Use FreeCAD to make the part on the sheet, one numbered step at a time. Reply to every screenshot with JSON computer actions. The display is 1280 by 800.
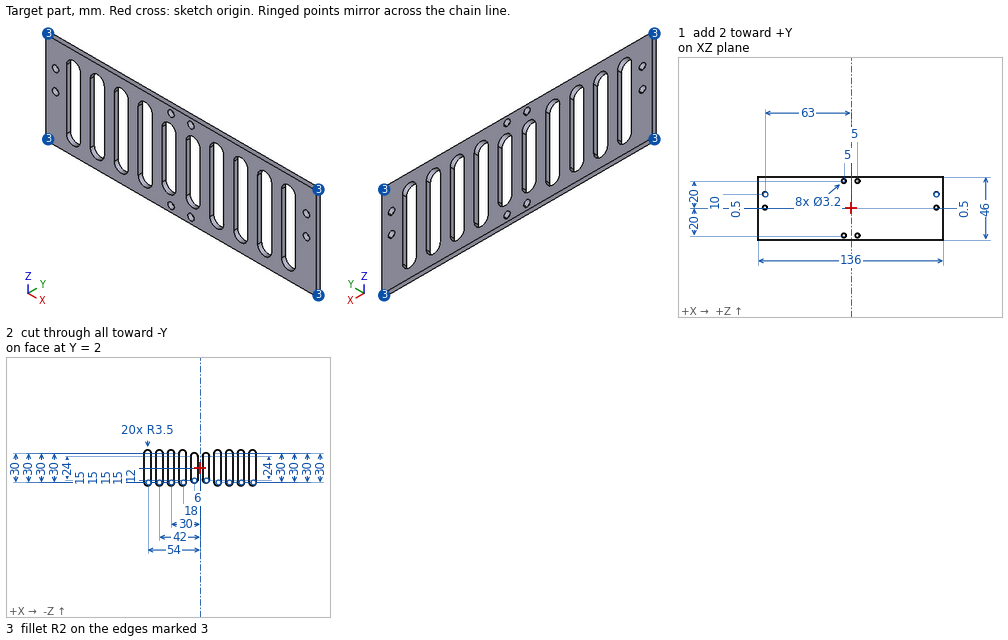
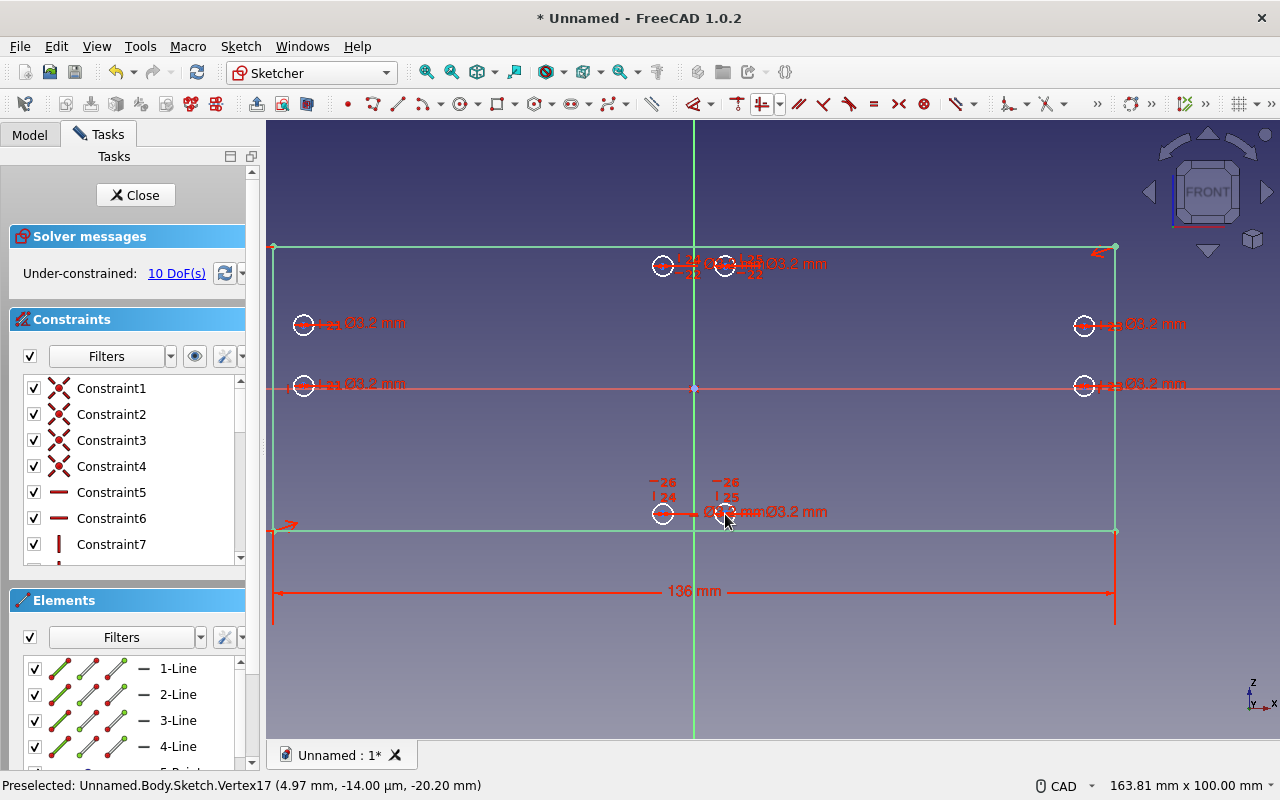
{"action": "left_click", "coordinate": [304, 325]}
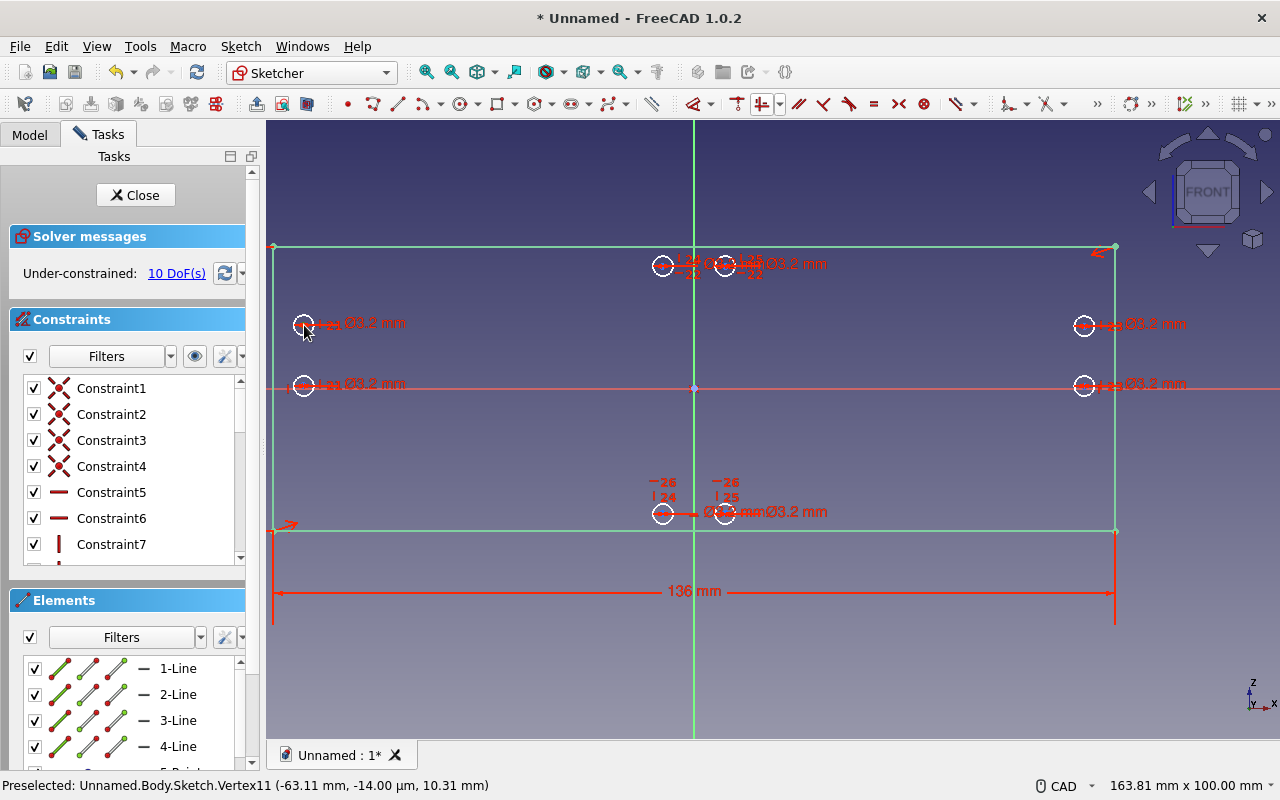
{"action": "left_click", "coordinate": [1084, 326]}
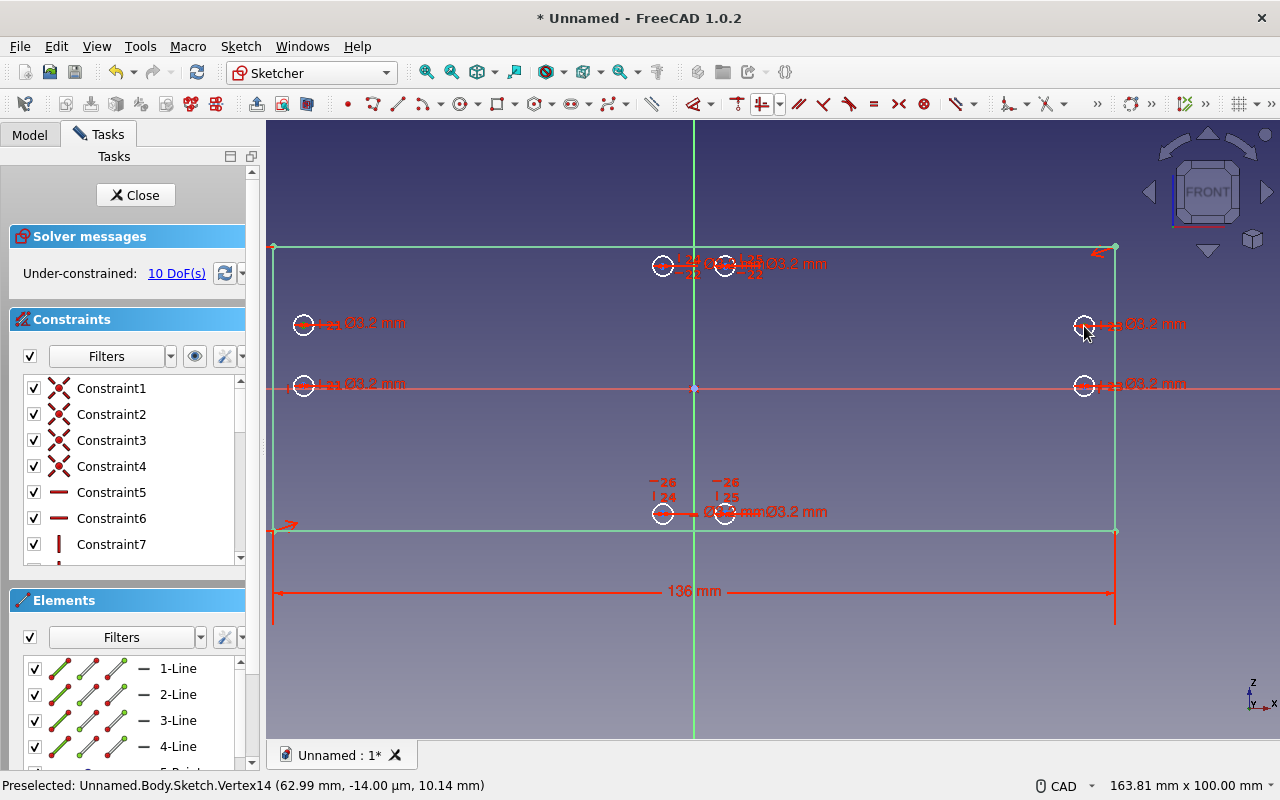
{"action": "left_click", "coordinate": [694, 671]}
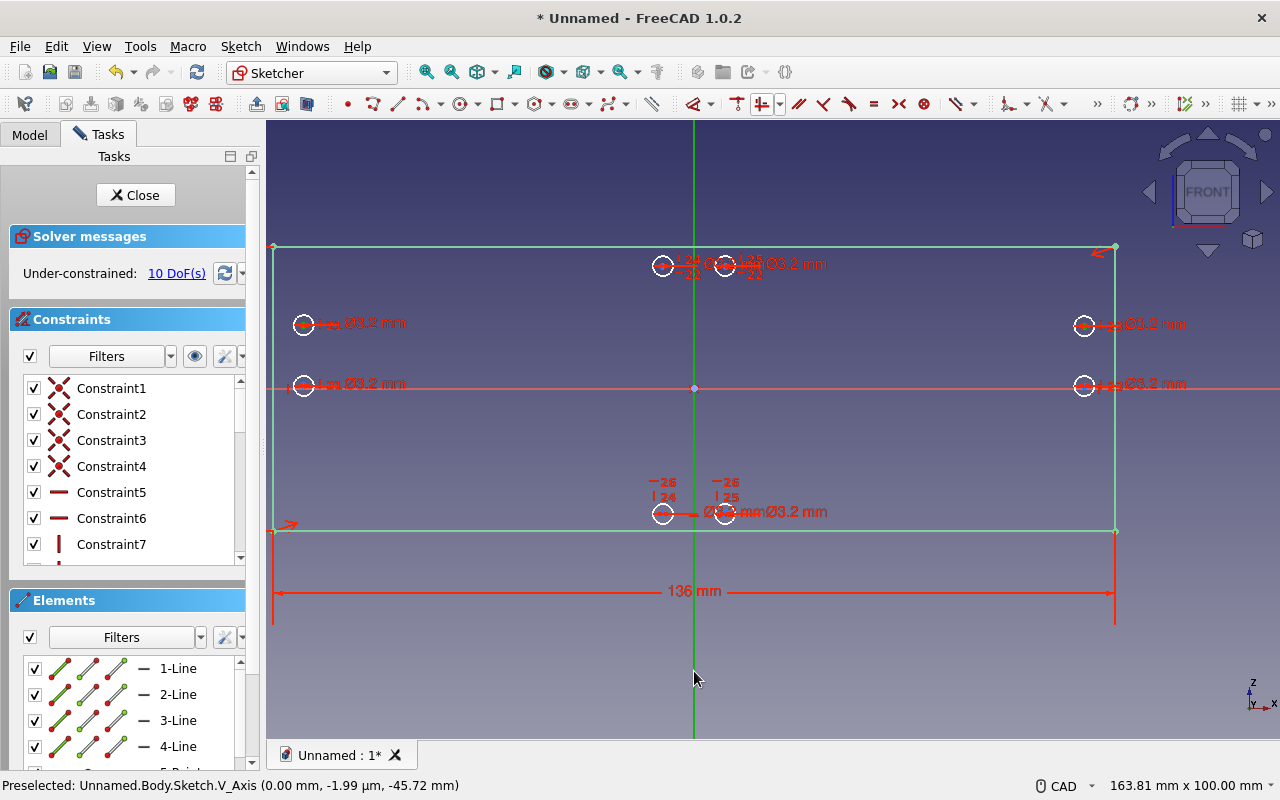
{"action": "left_click", "coordinate": [899, 104]}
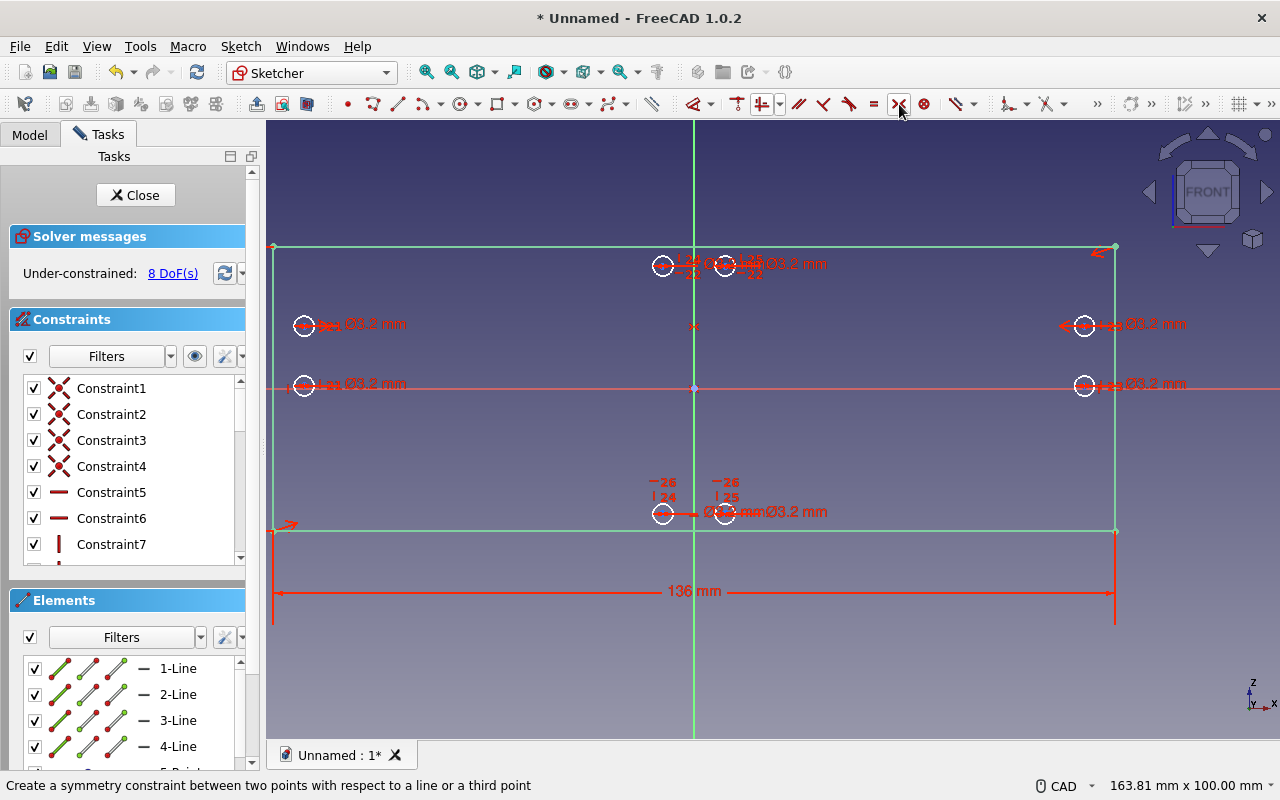
{"action": "left_click", "coordinate": [692, 104]}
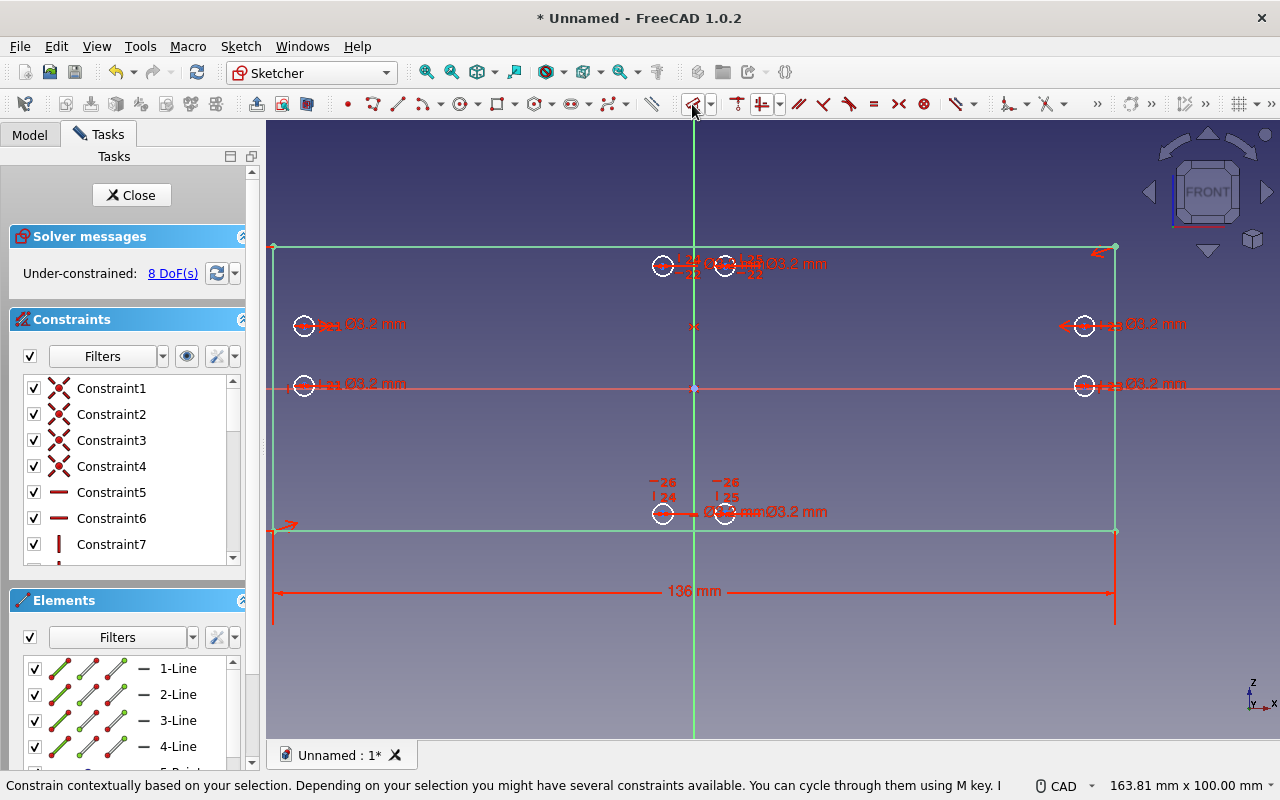
{"action": "scroll", "coordinate": [663, 266], "scroll_direction": "up", "scroll_amount": 2}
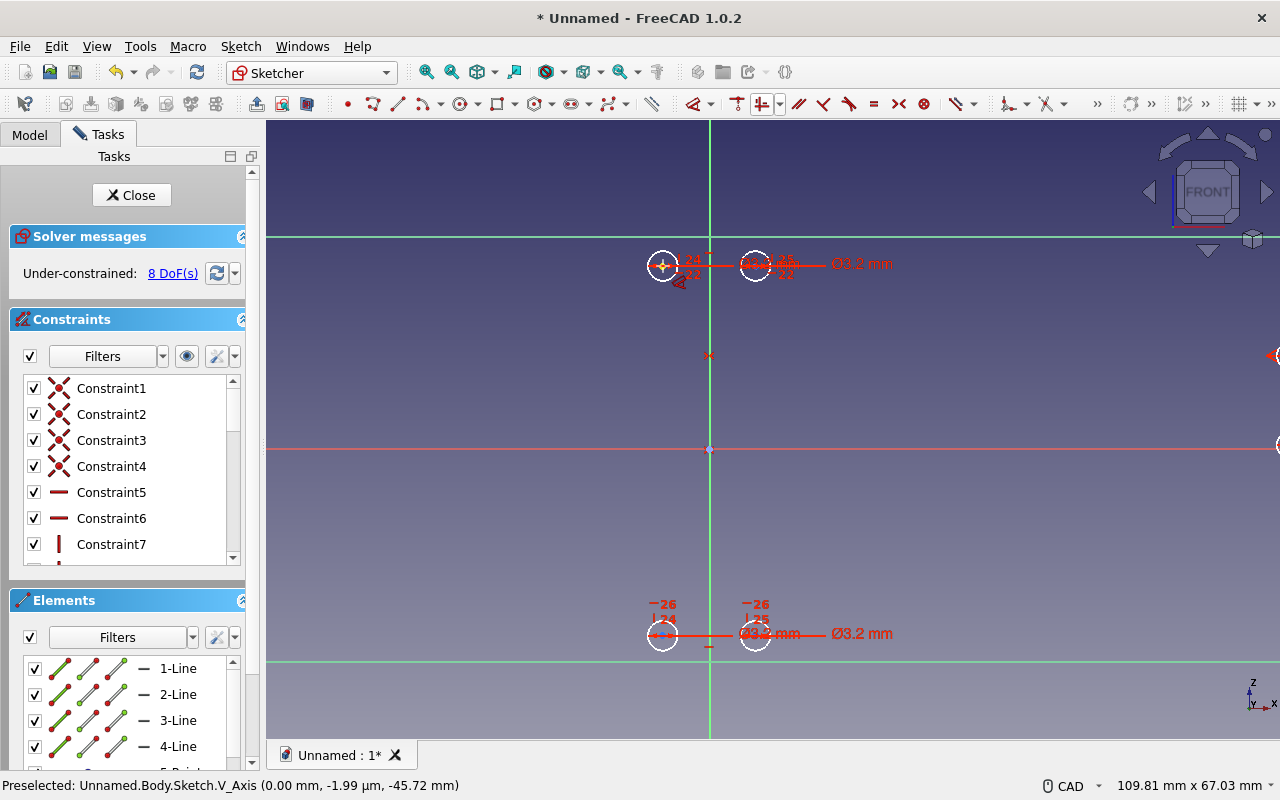
{"action": "left_click", "coordinate": [663, 266]}
{"action": "left_click", "coordinate": [686, 483]}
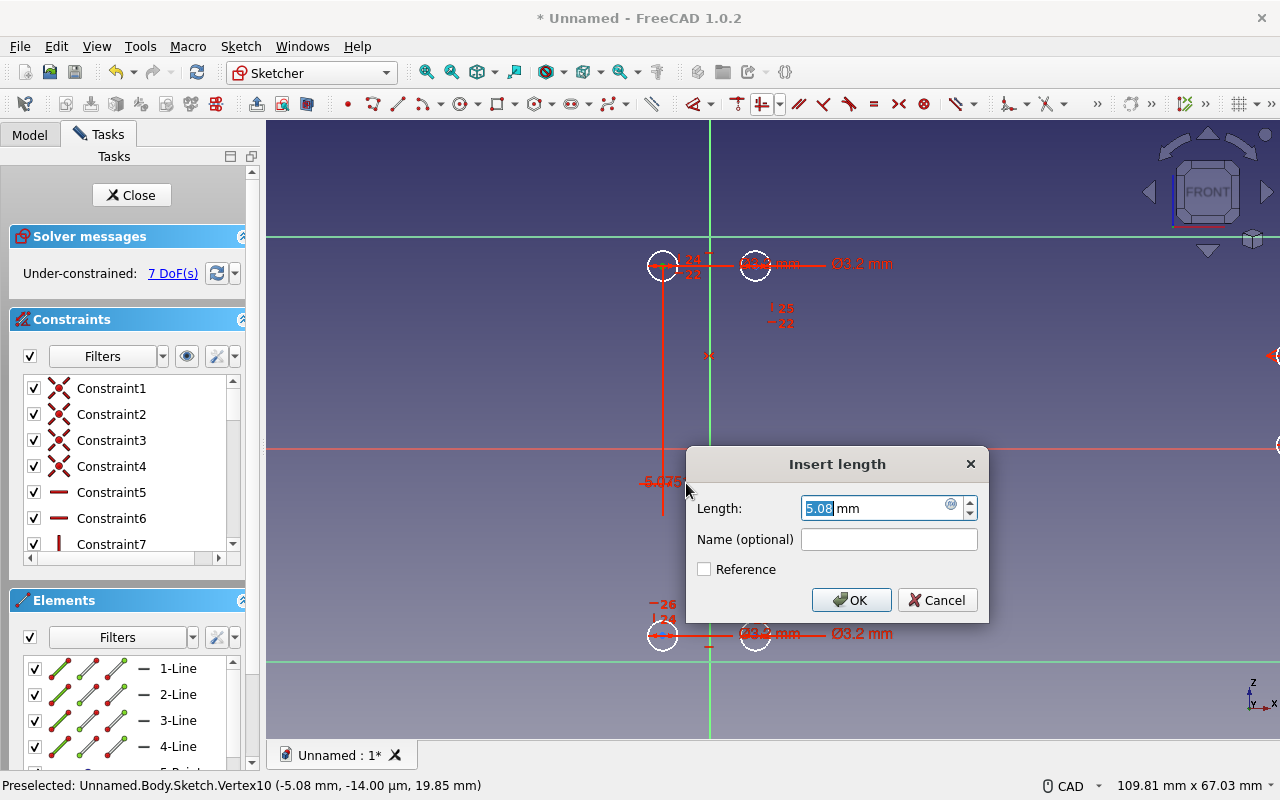
{"action": "type", "text": "5"}
{"action": "key", "text": "Return"}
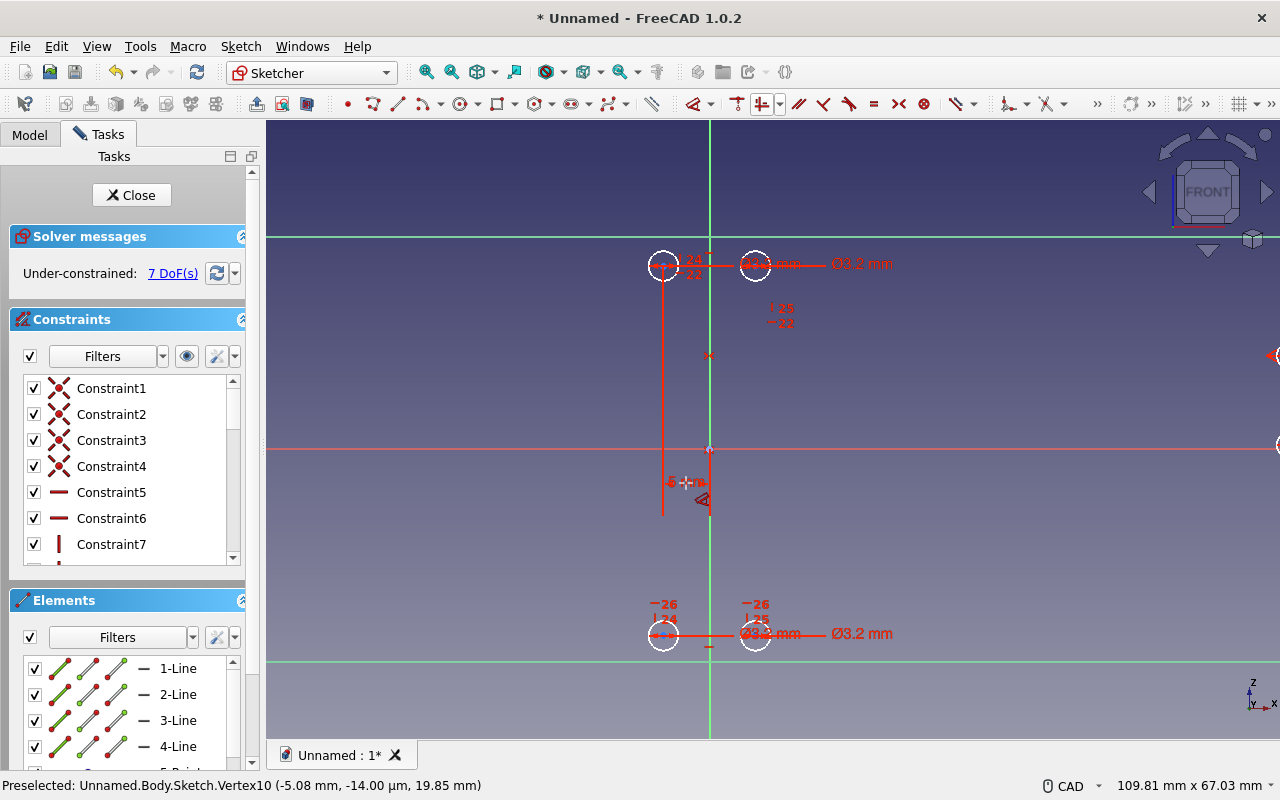
{"action": "left_click", "coordinate": [756, 266]}
{"action": "left_click", "coordinate": [733, 208]}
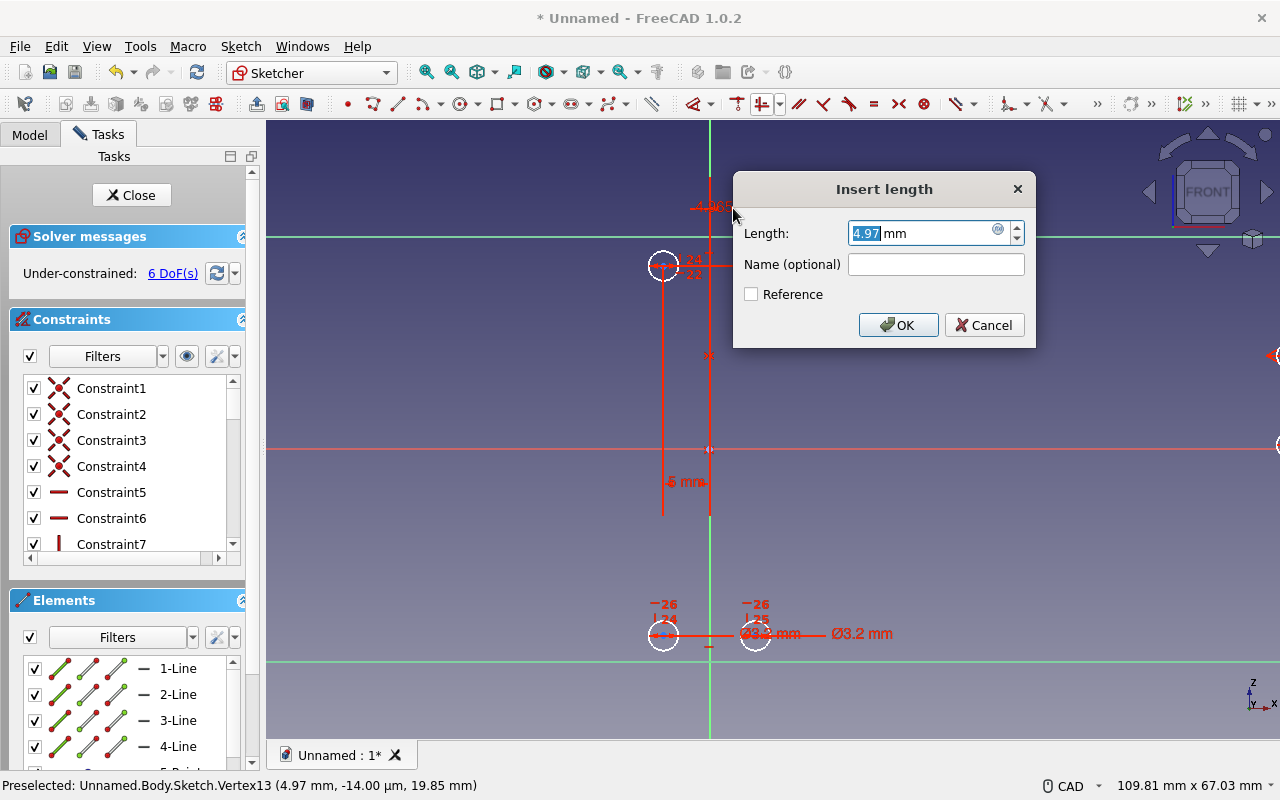
{"action": "type", "text": "5"}
{"action": "key", "text": "Return"}